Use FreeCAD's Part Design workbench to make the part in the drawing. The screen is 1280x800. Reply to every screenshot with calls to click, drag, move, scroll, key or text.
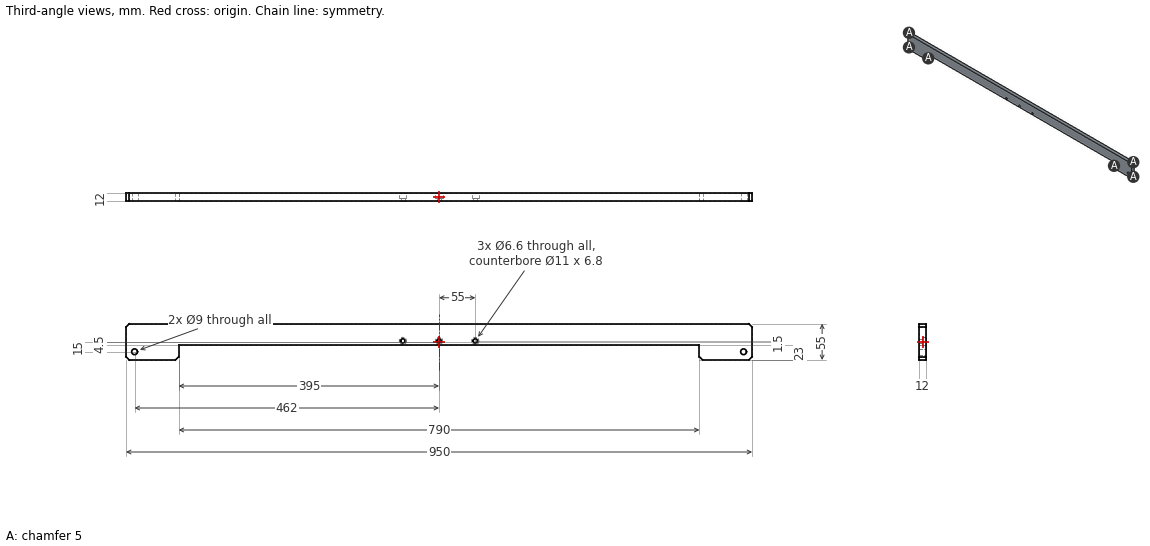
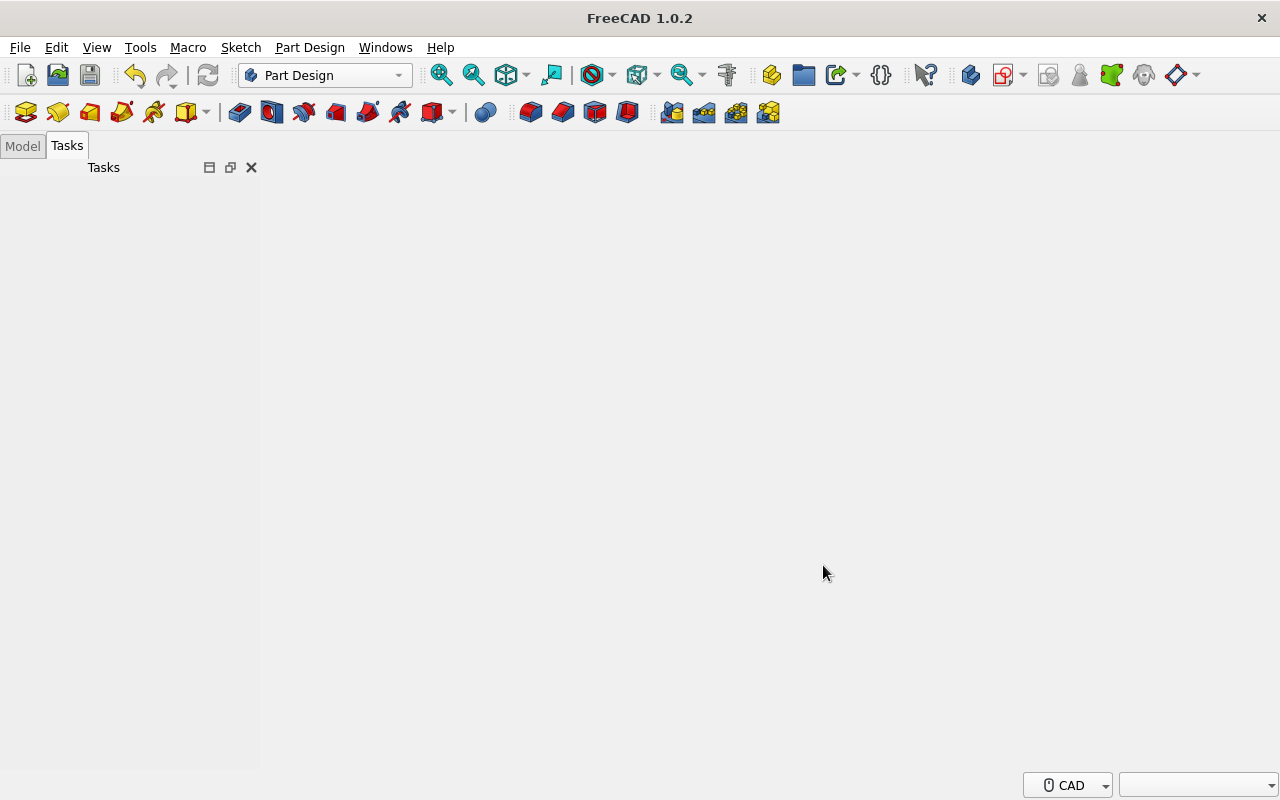
key(ctrl+n)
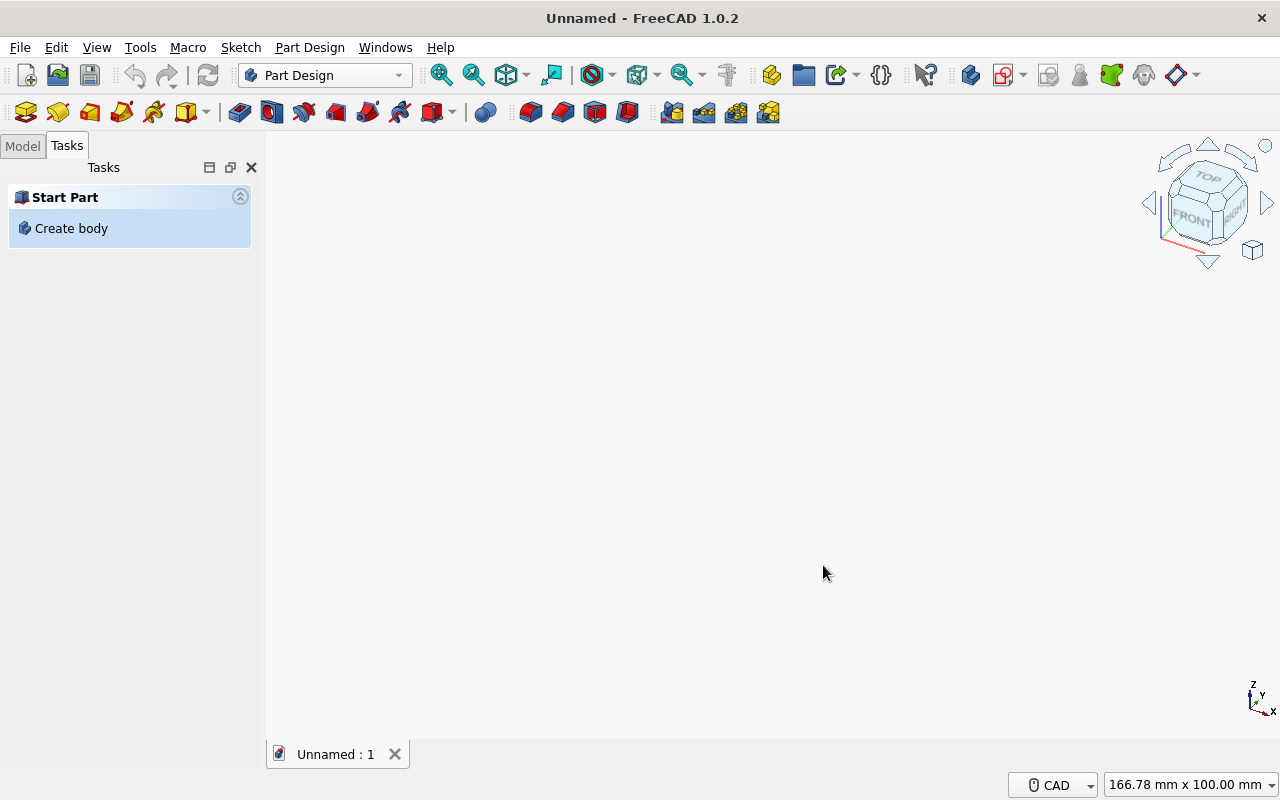
click(1004, 76)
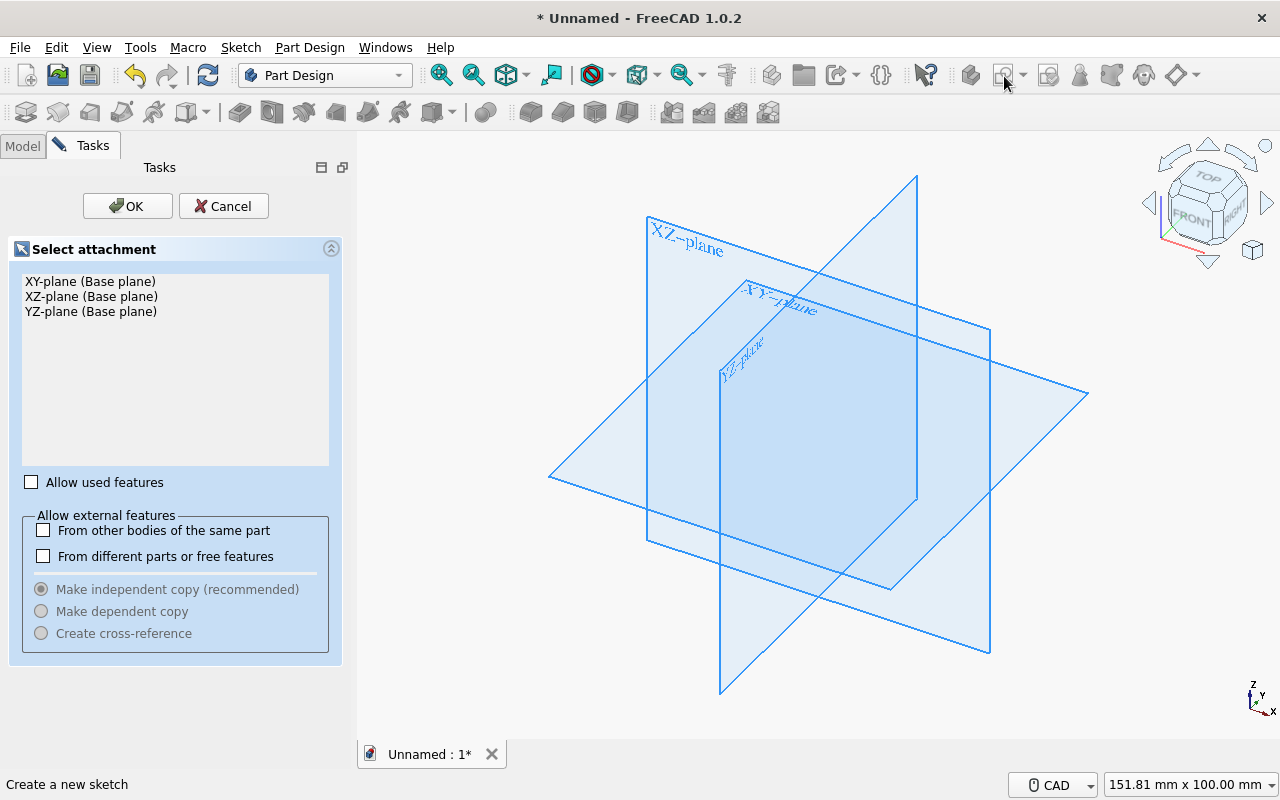
click(82, 296)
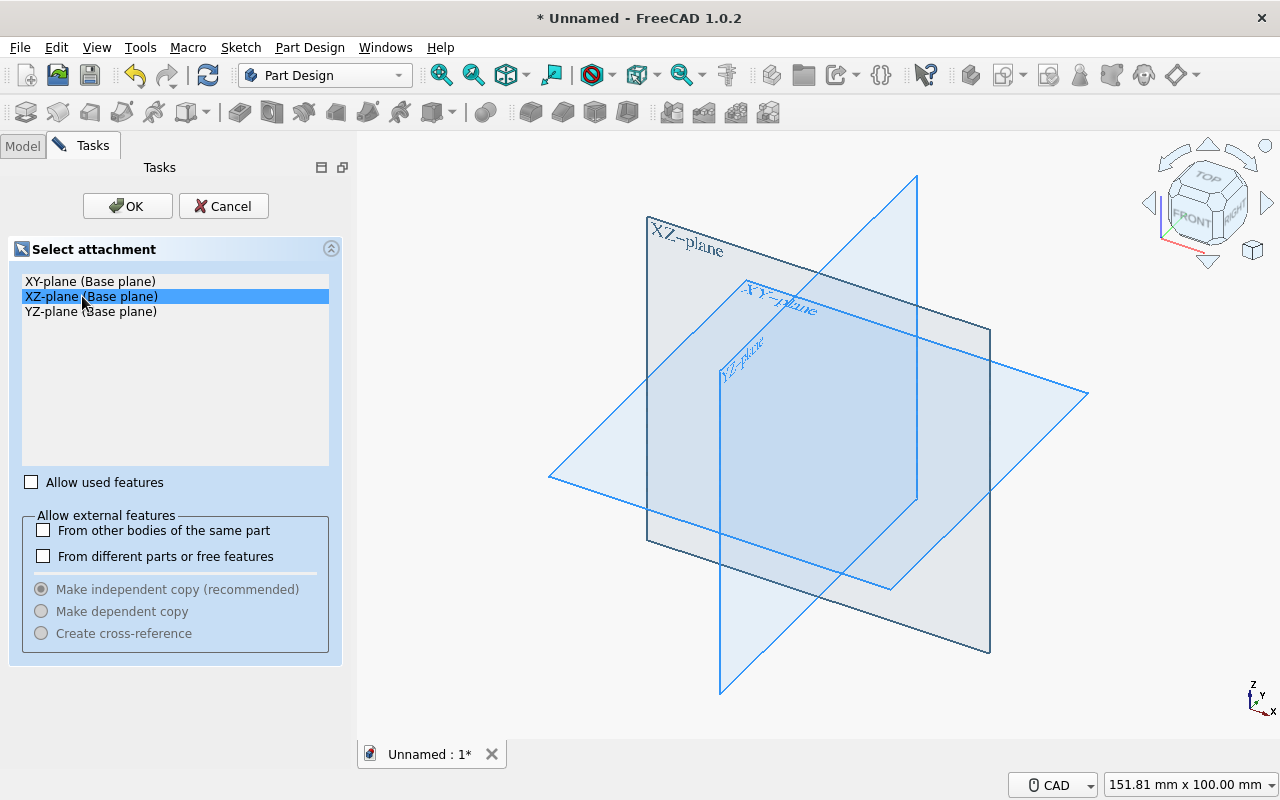
click(128, 206)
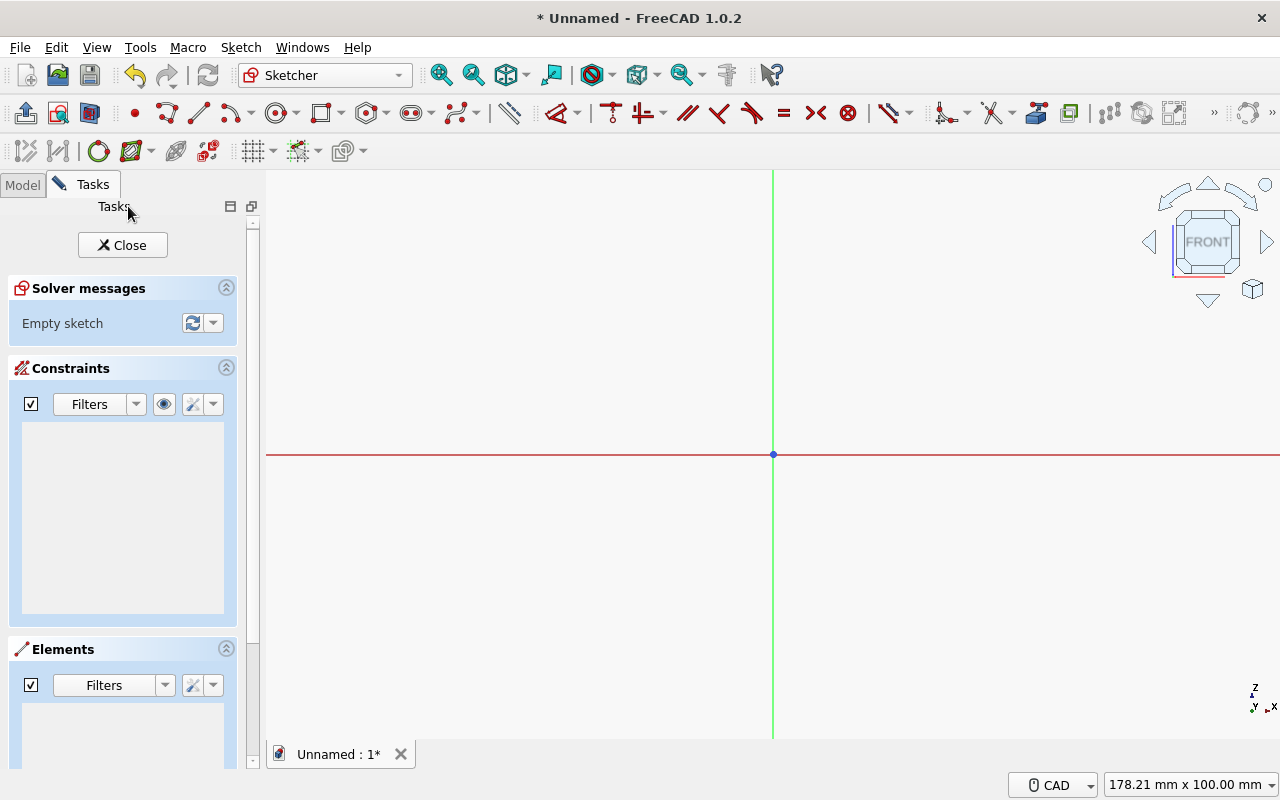
scroll(696, 454, down, 11)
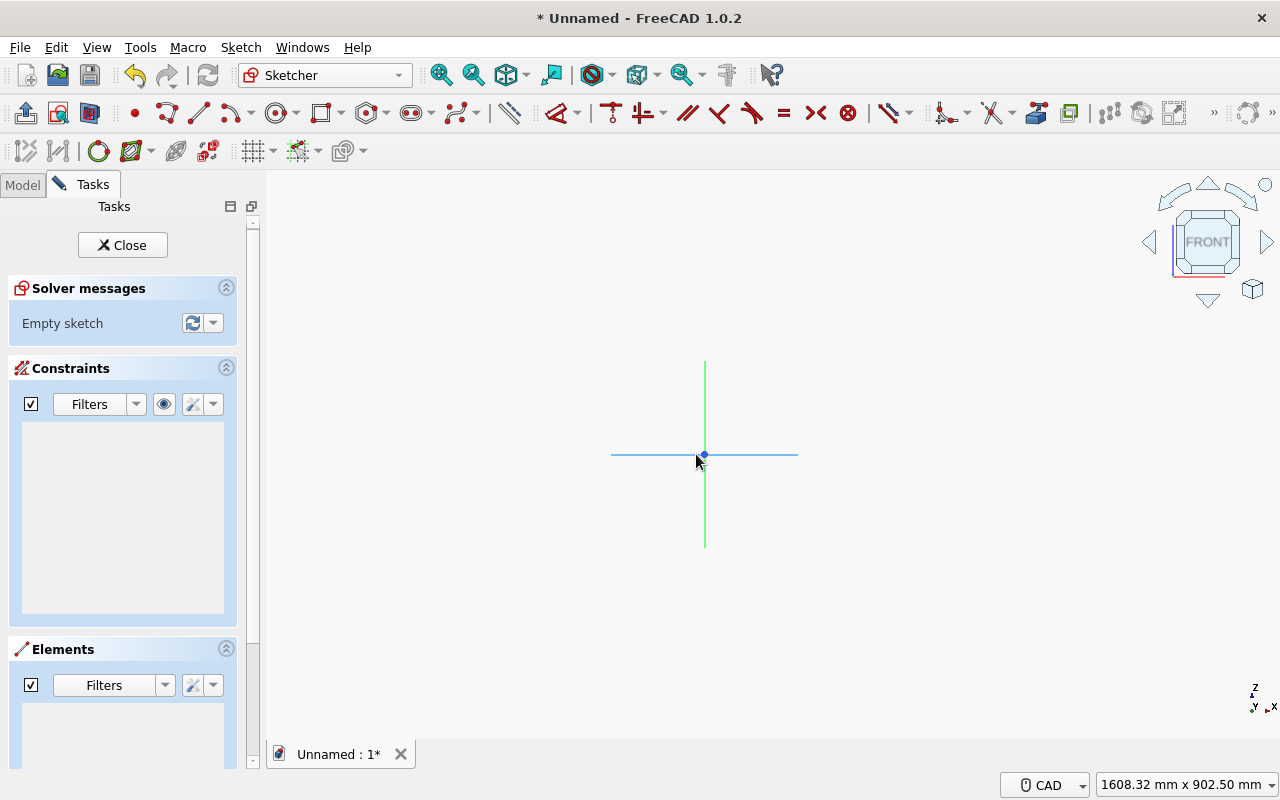
click(344, 114)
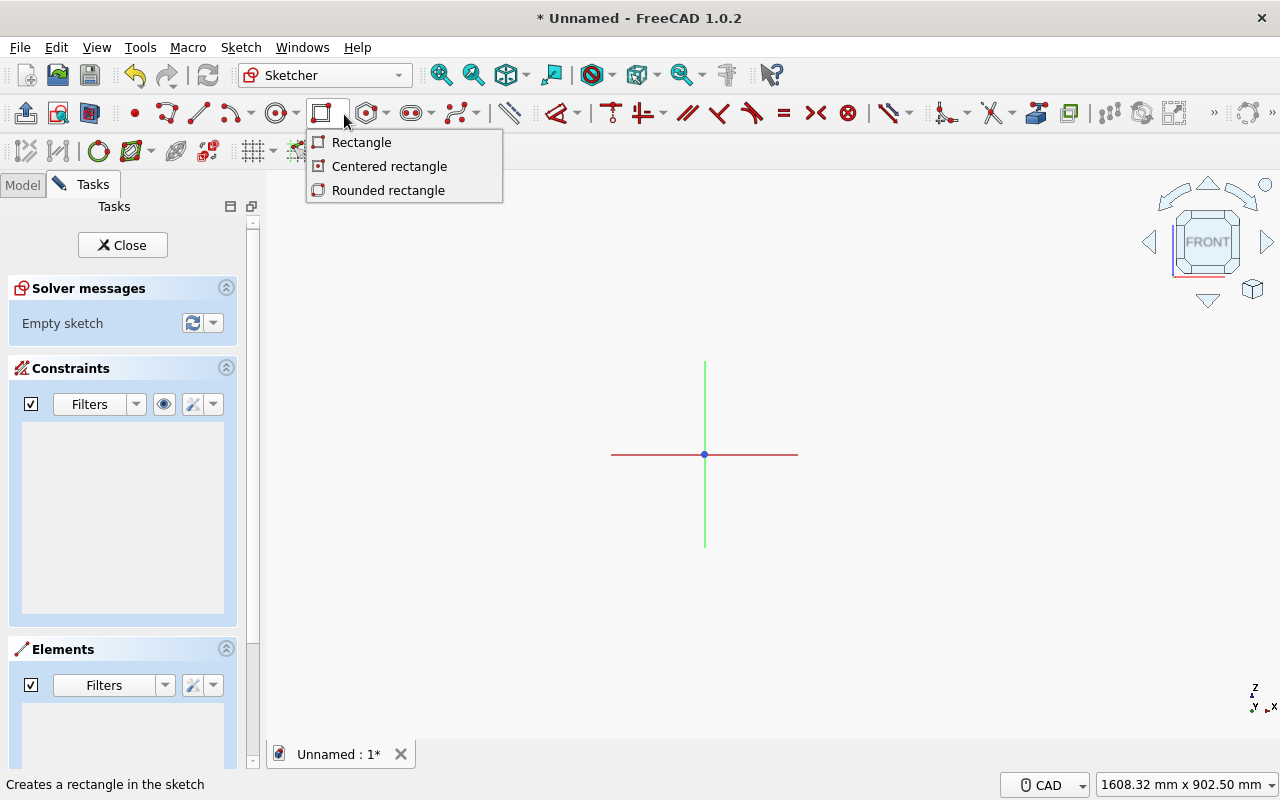
click(404, 166)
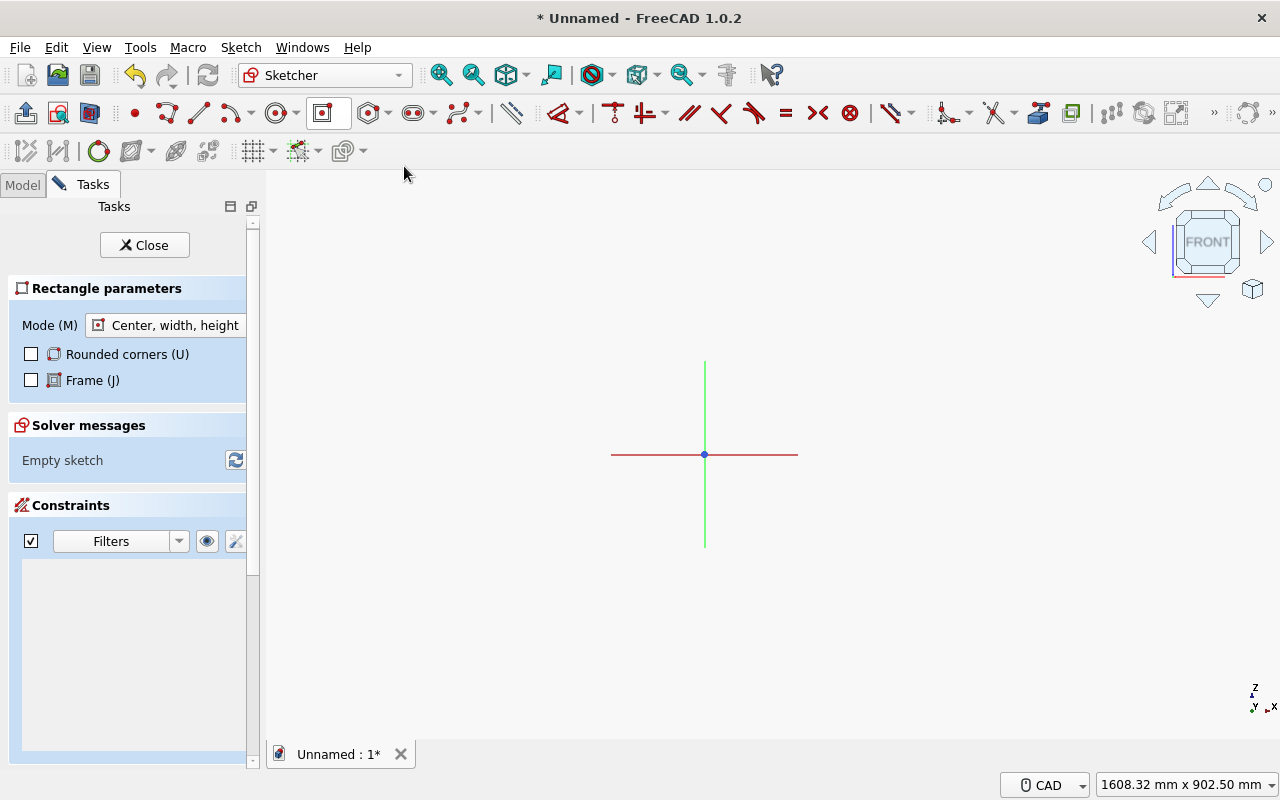
click(705, 454)
move(1004, 437)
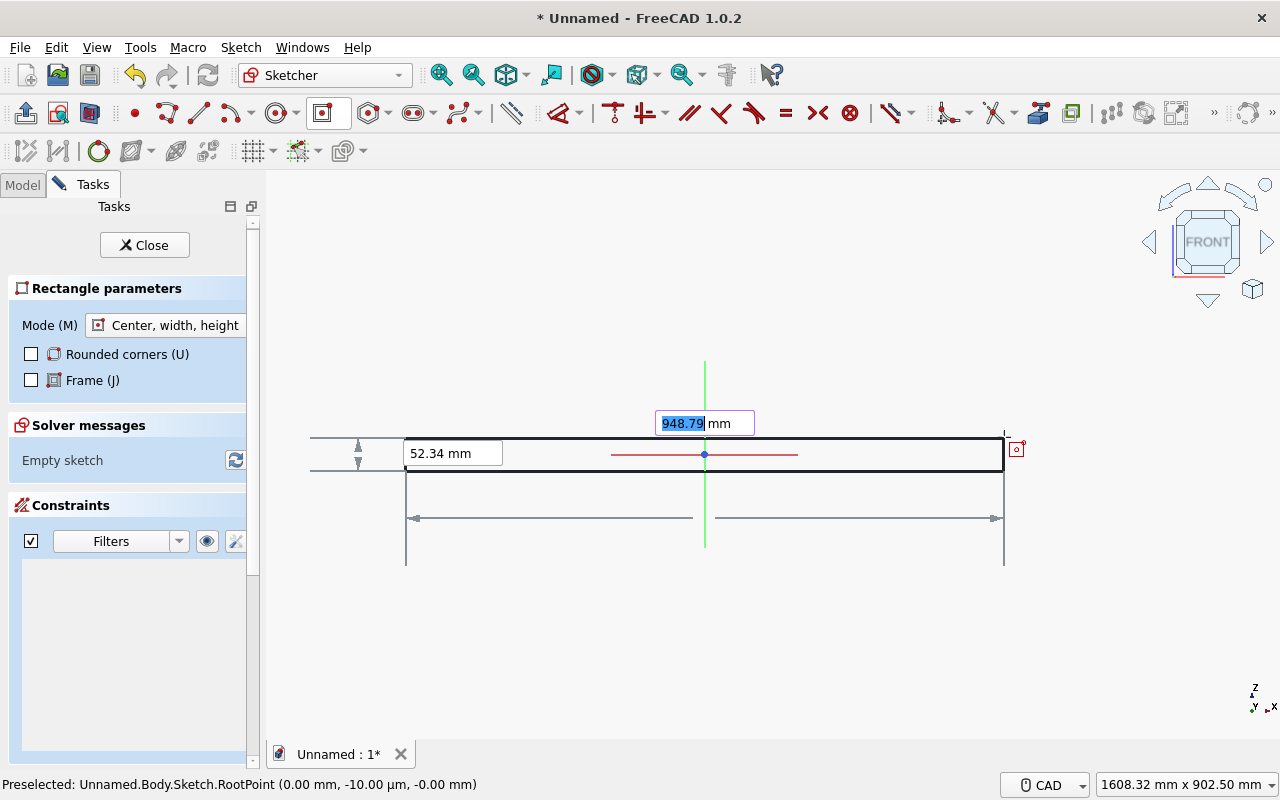
text(950)
key(Tab)
text(55)
key(Return)
key(Escape)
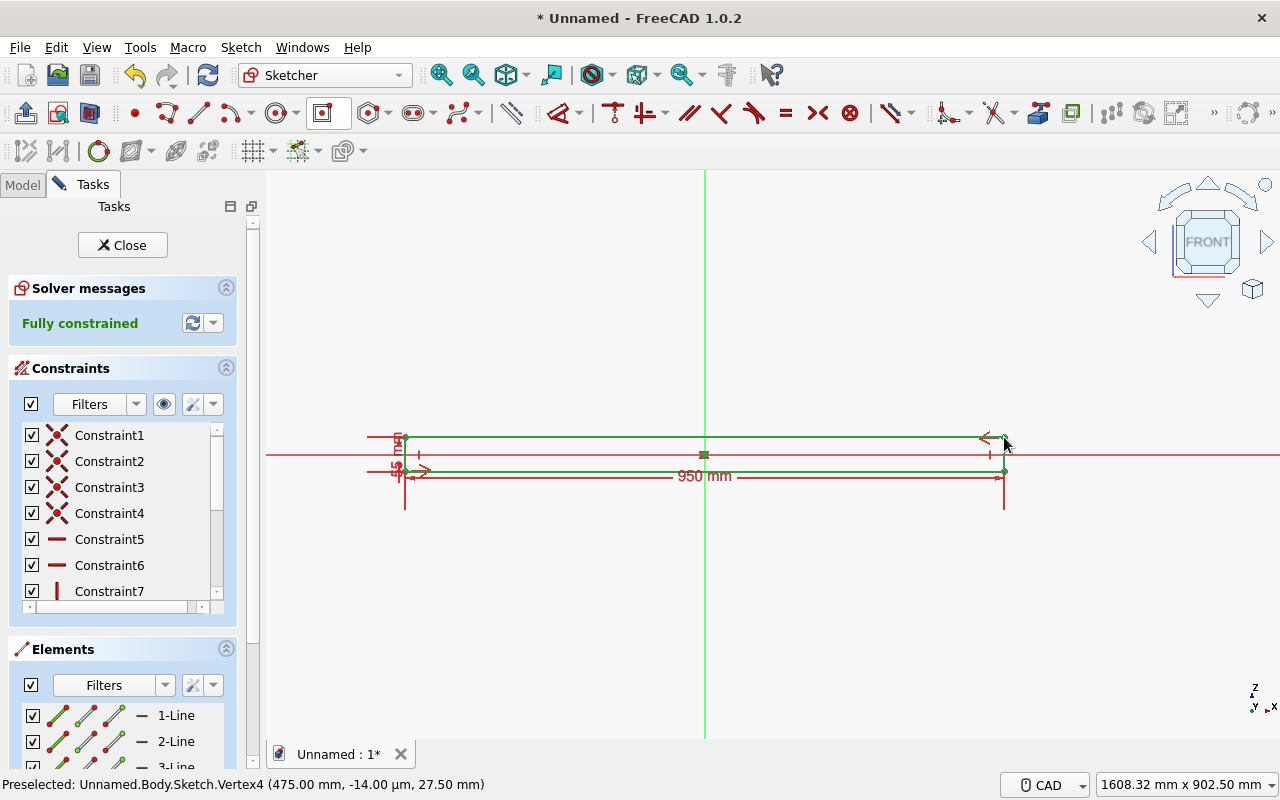
click(123, 245)